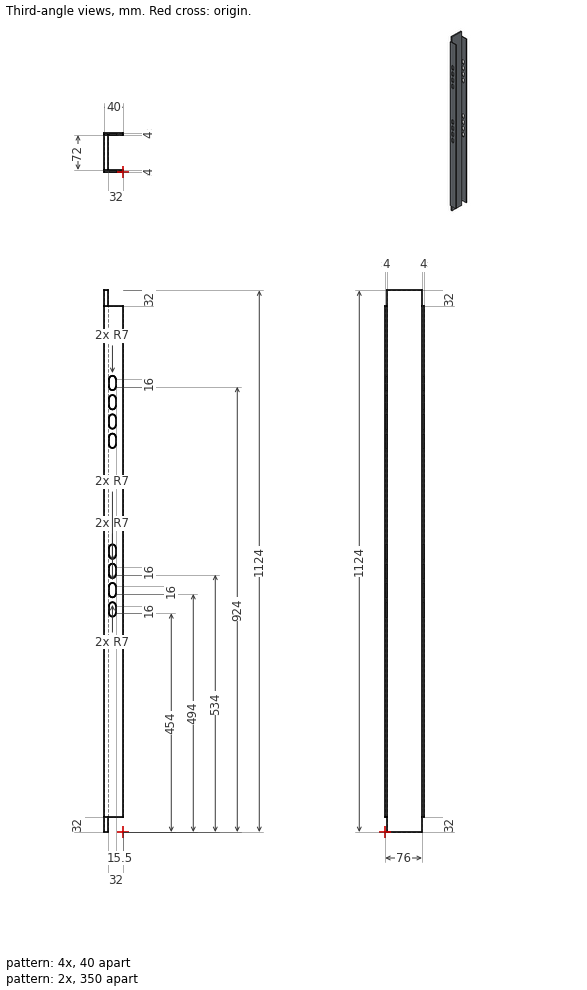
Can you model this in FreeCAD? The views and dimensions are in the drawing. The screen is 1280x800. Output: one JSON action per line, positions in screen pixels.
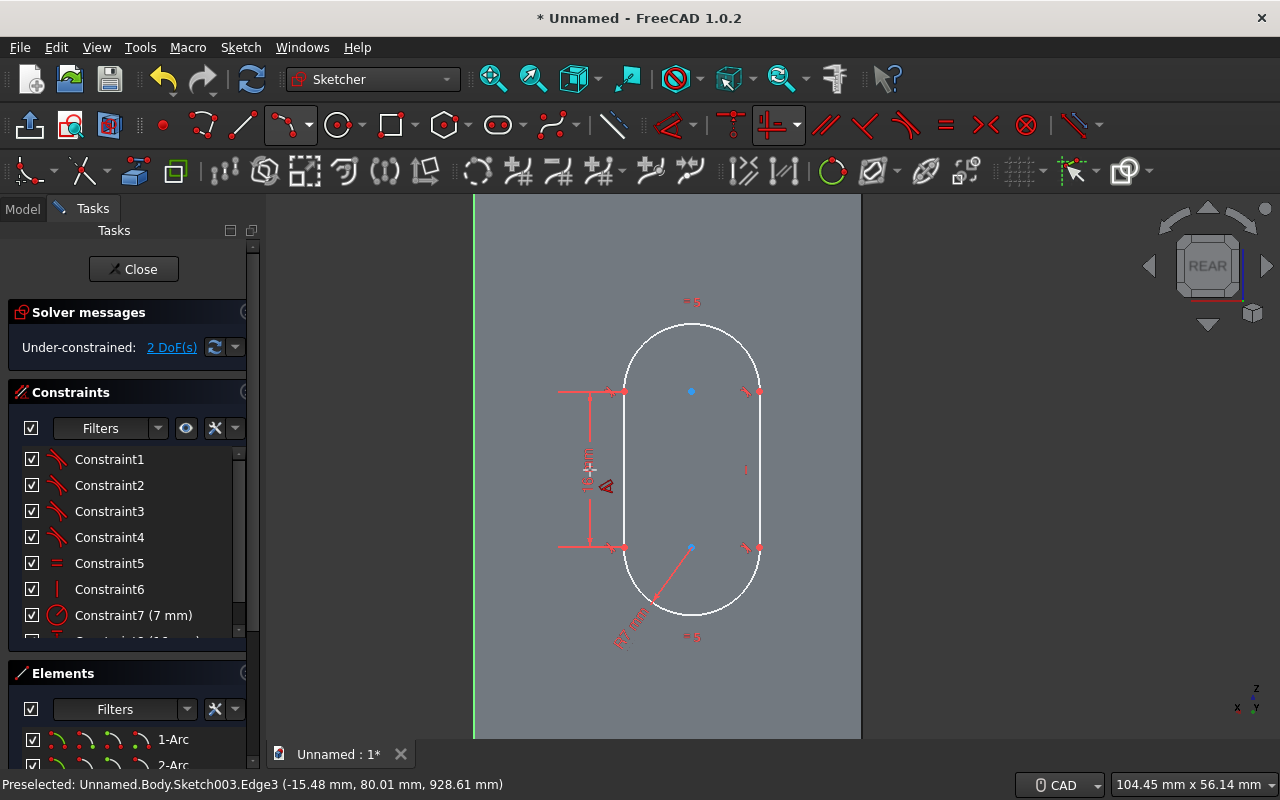
{"action": "left_click", "coordinate": [624, 547]}
{"action": "left_click", "coordinate": [440, 629]}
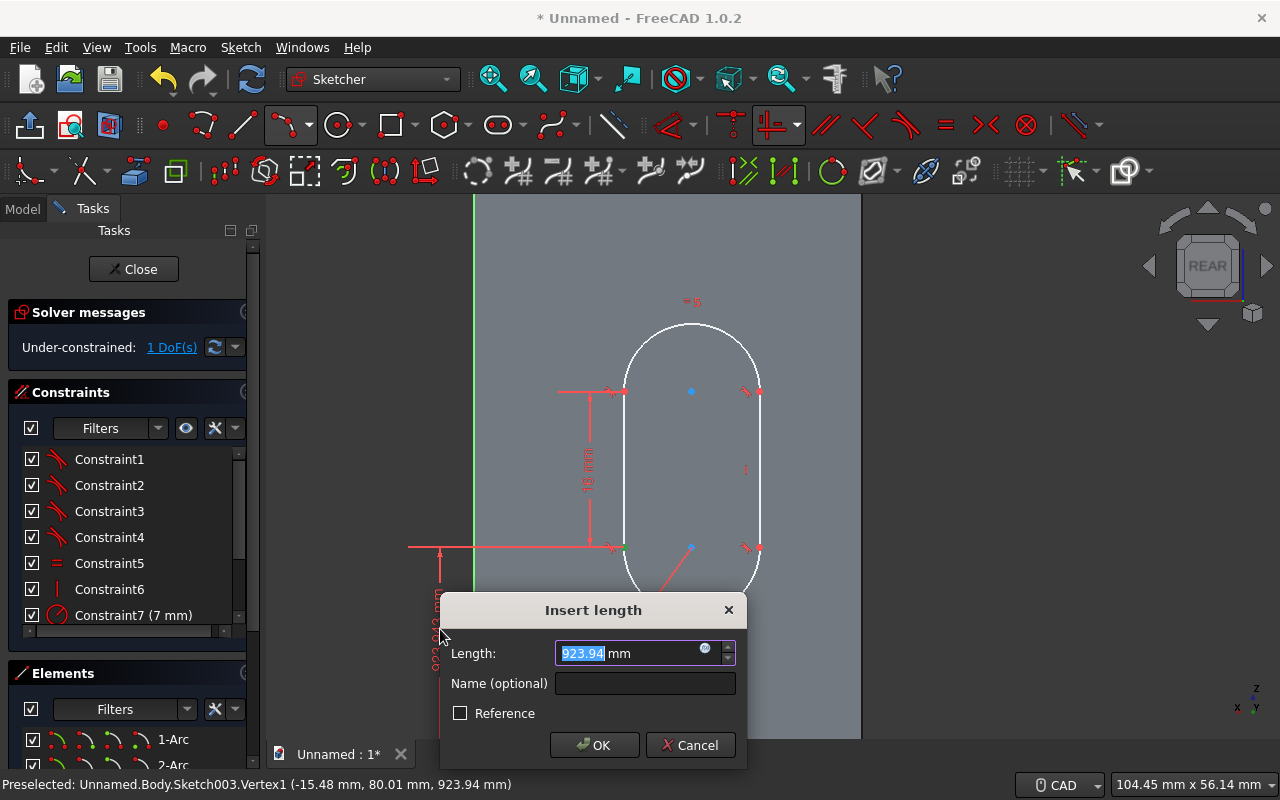
{"action": "type", "text": "924"}
{"action": "key", "text": "Return"}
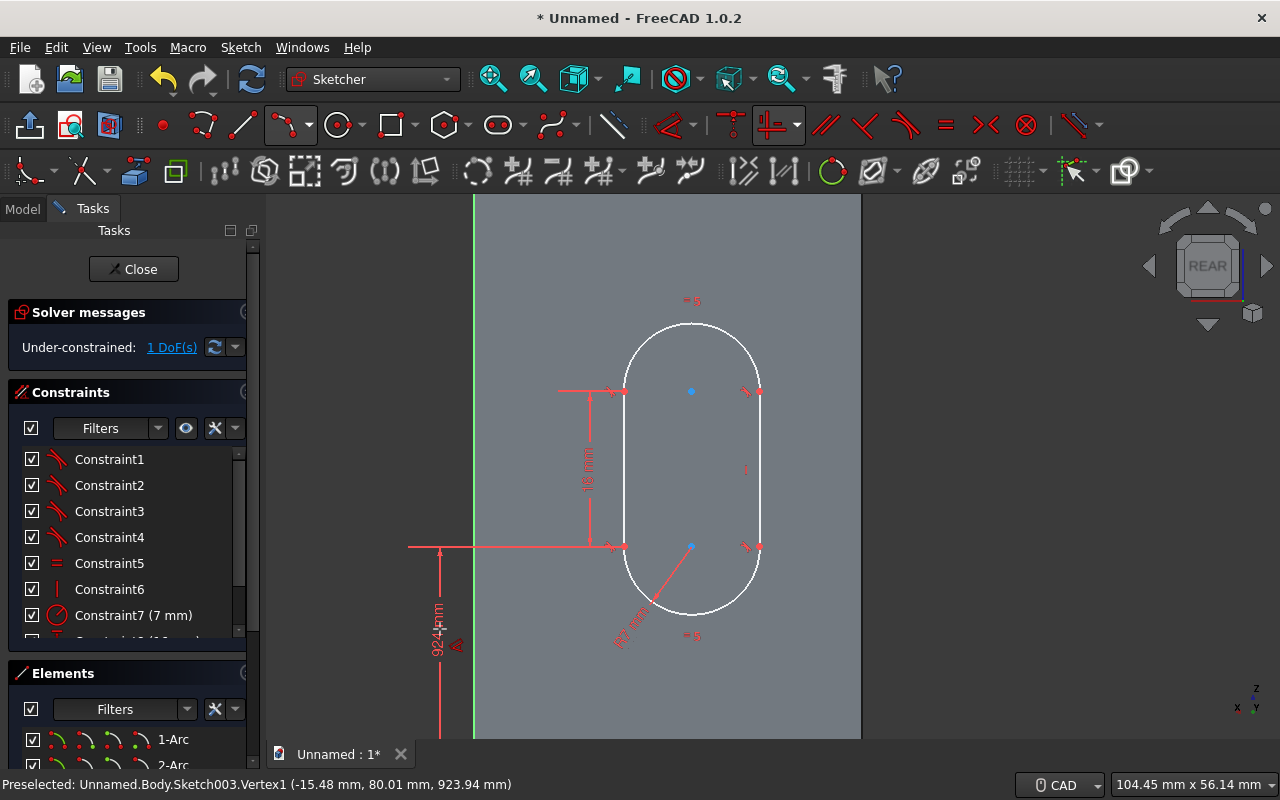
{"action": "left_click", "coordinate": [624, 547]}
{"action": "left_click", "coordinate": [549, 513]}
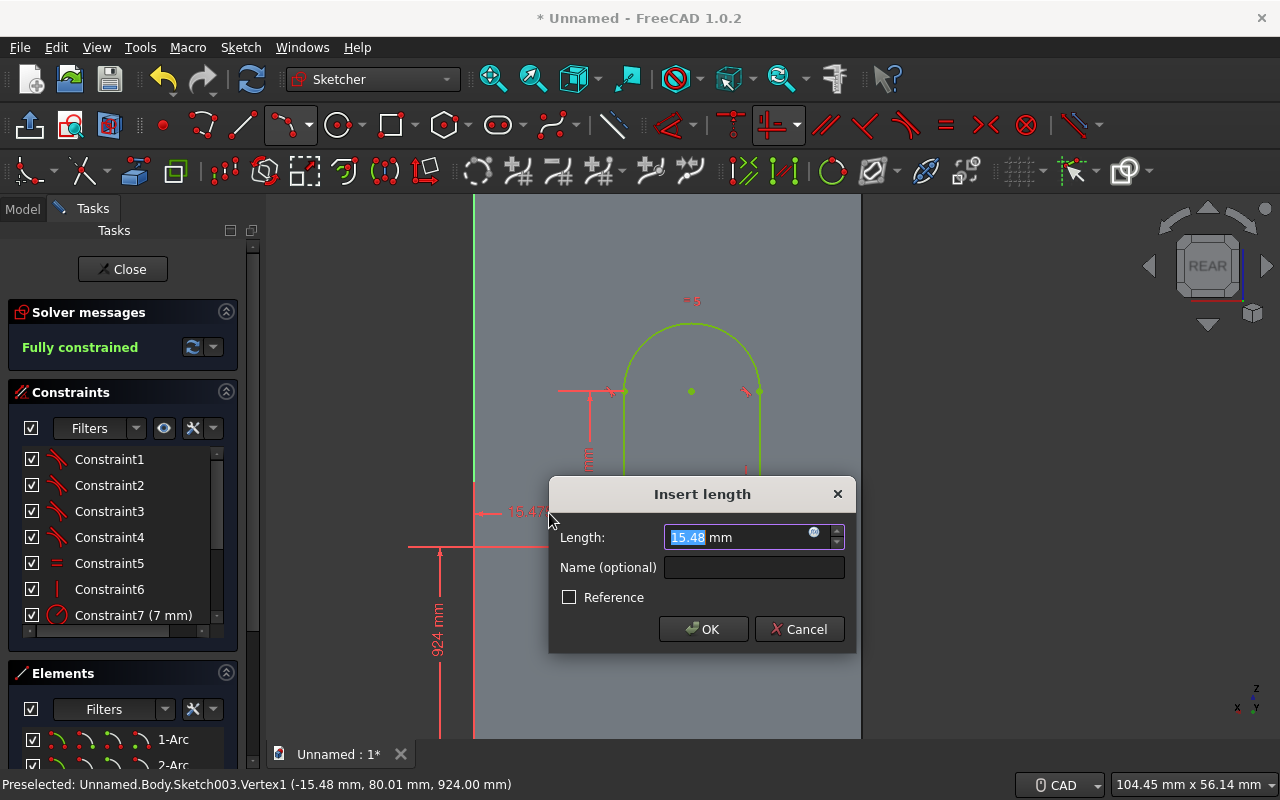
{"action": "type", "text": "15.5"}
{"action": "key", "text": "Return"}
{"action": "key", "text": "Escape"}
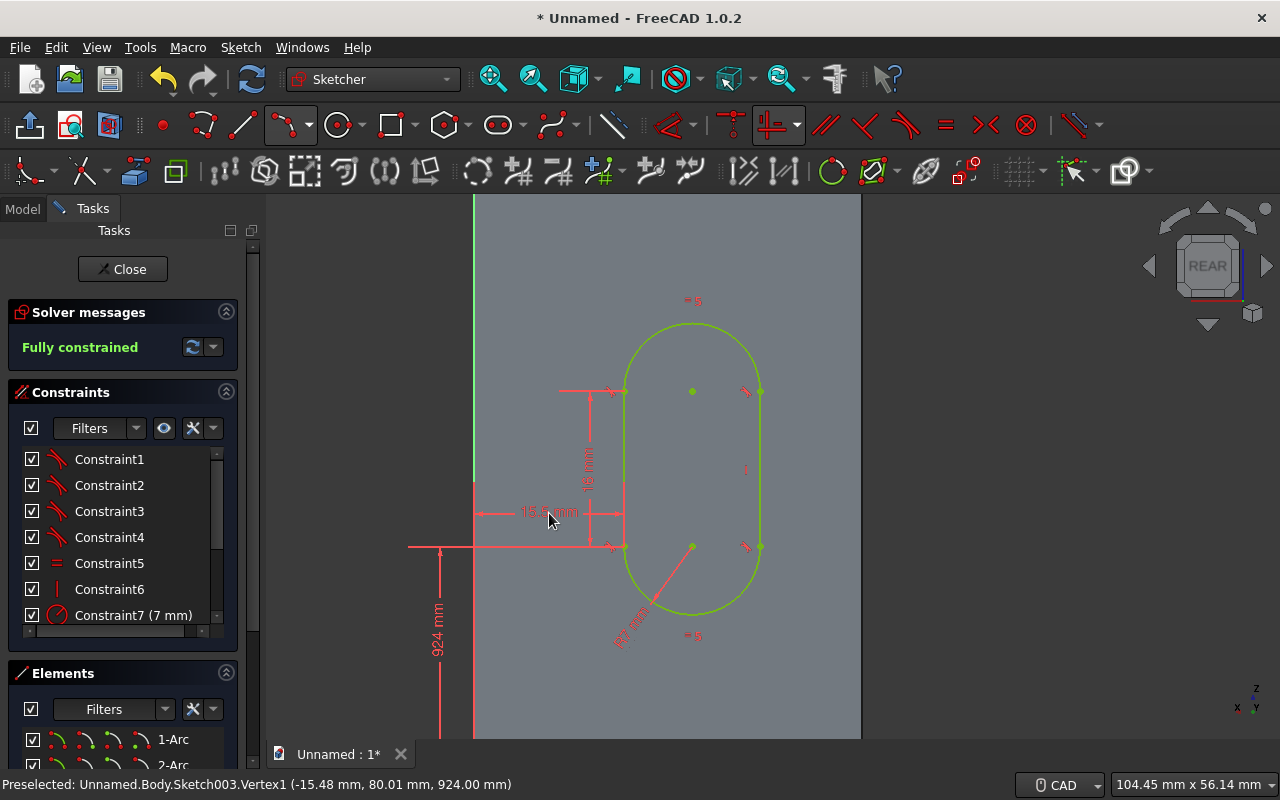
{"action": "left_click", "coordinate": [123, 269]}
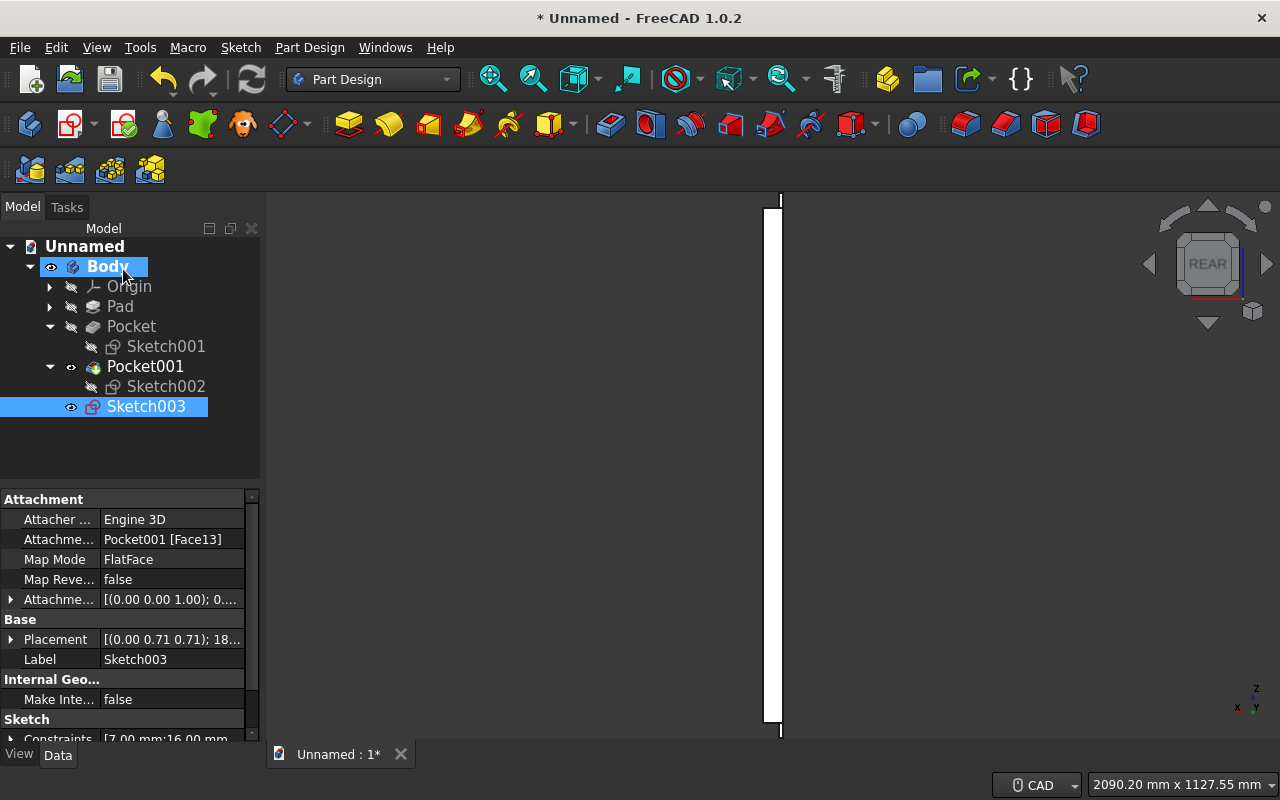
{"action": "left_click", "coordinate": [612, 124]}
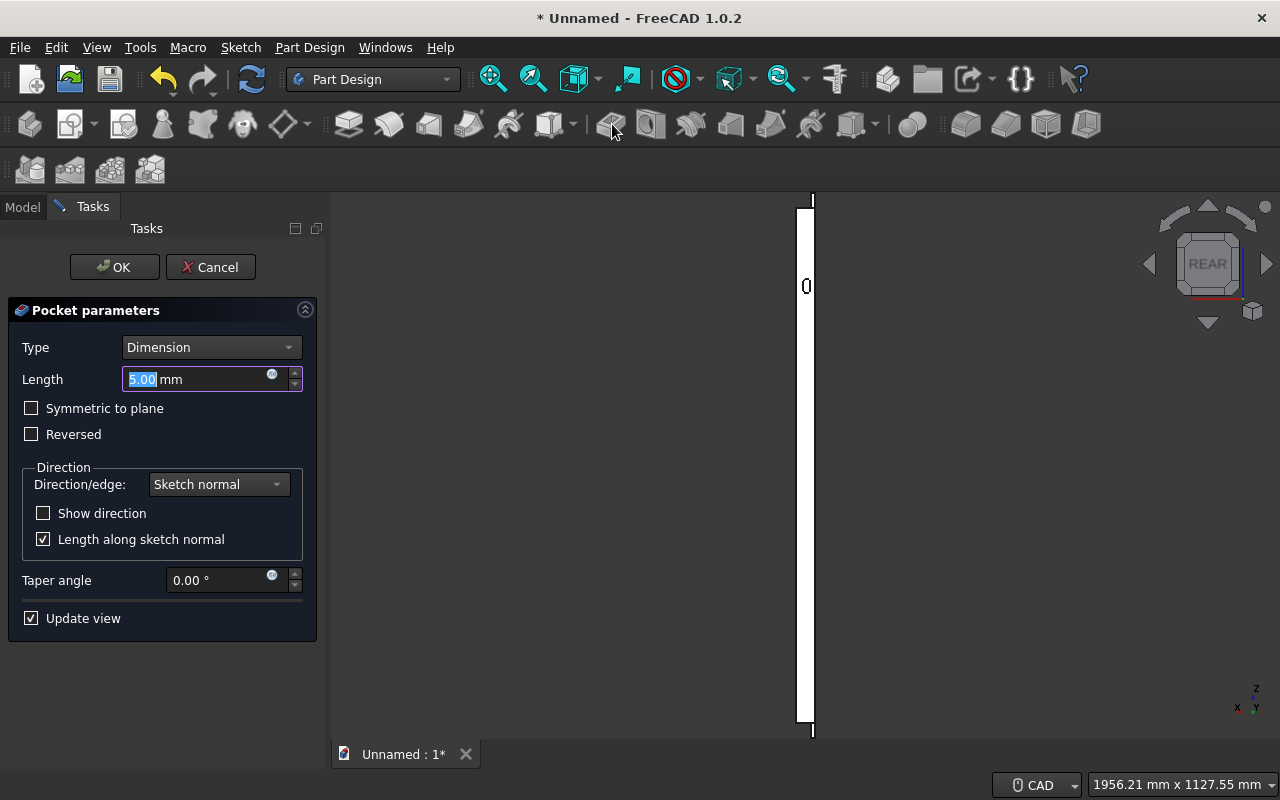
{"action": "left_click", "coordinate": [212, 348]}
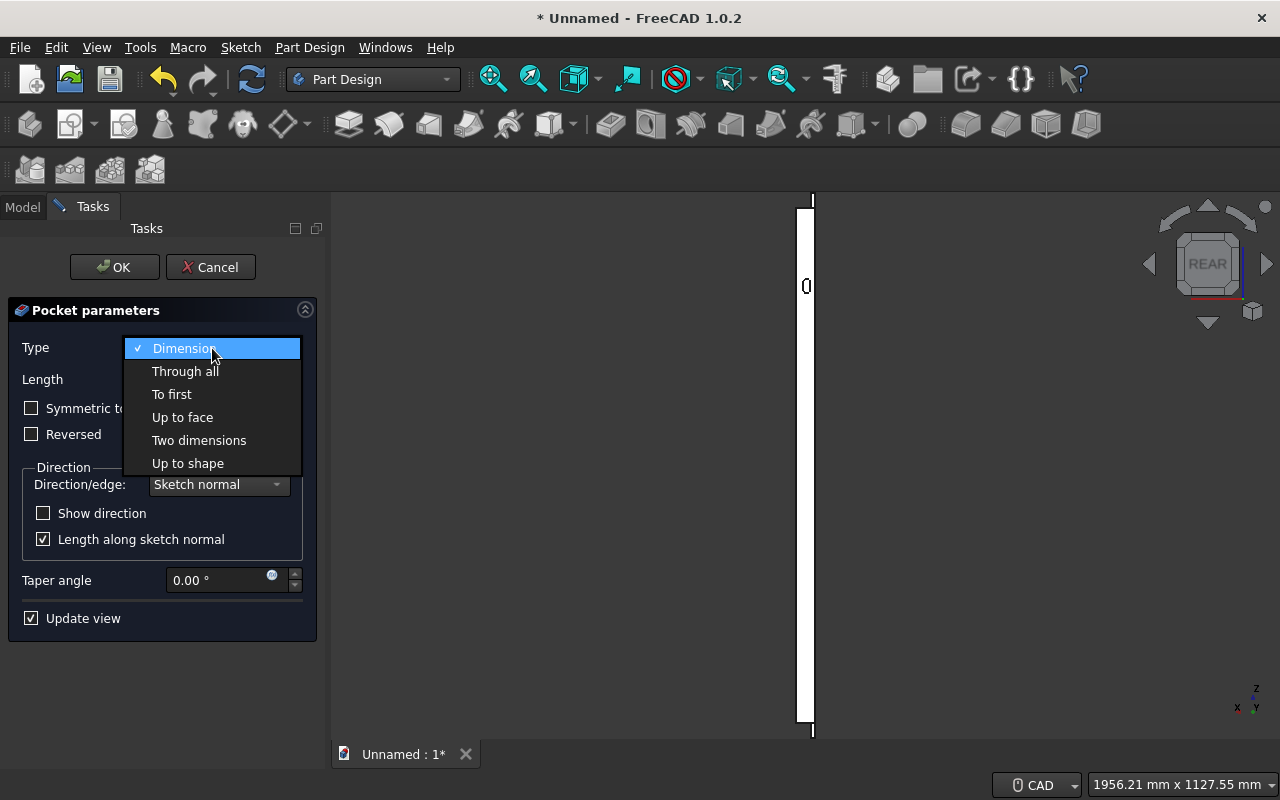
{"action": "left_click", "coordinate": [212, 372]}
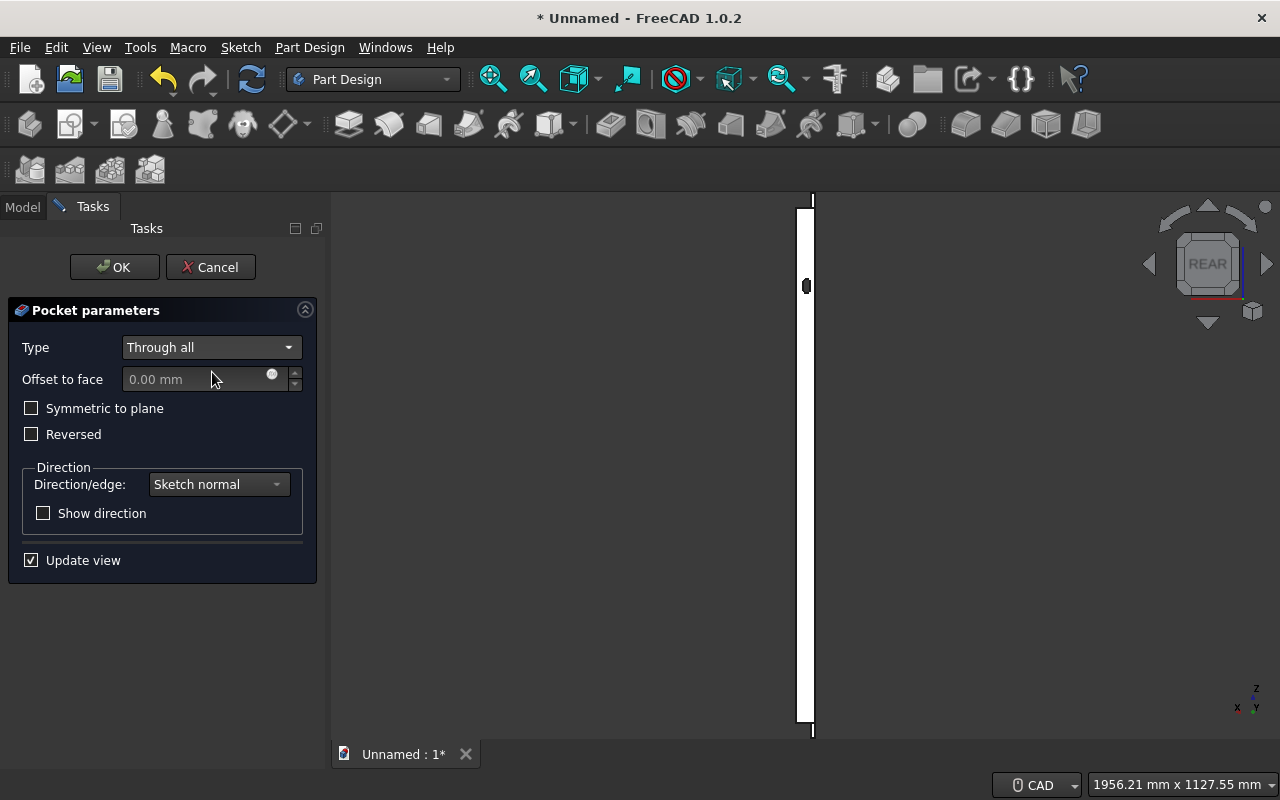
{"action": "left_click", "coordinate": [115, 267]}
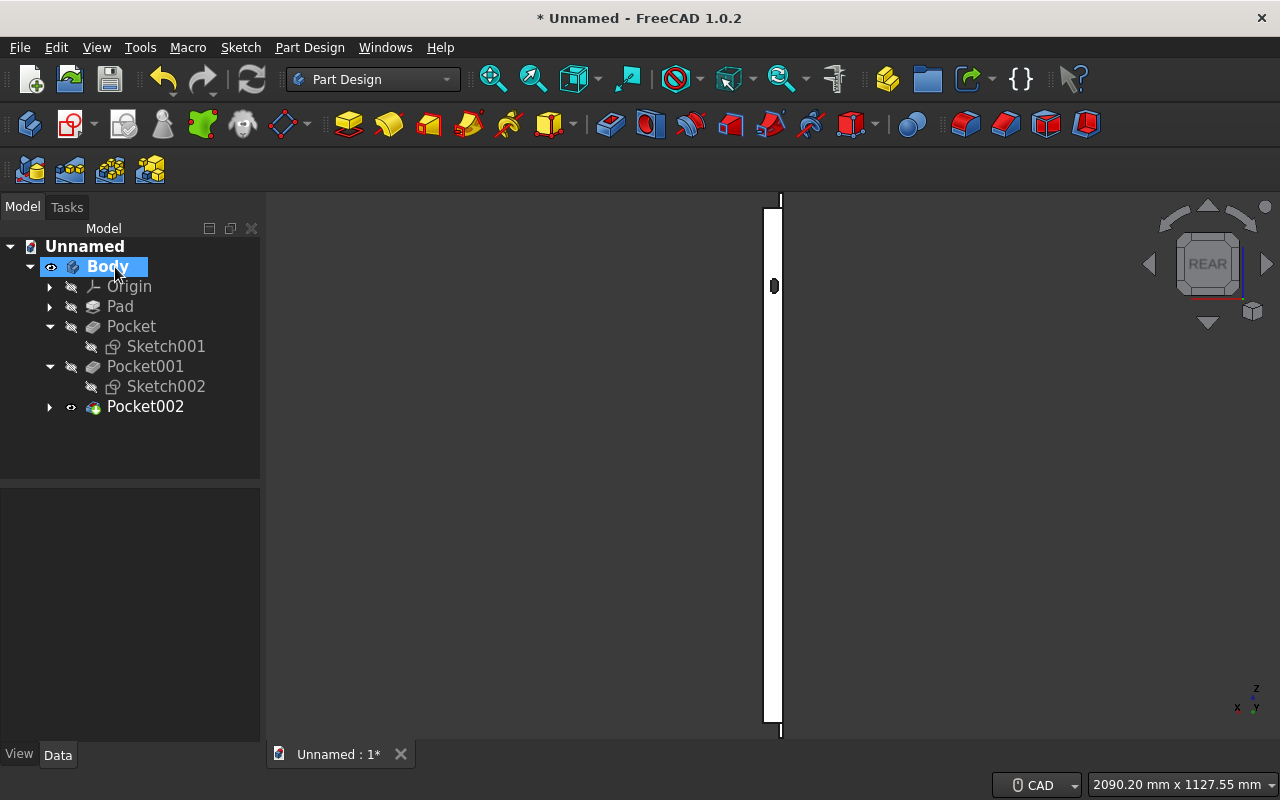
{"action": "left_click", "coordinate": [116, 407]}